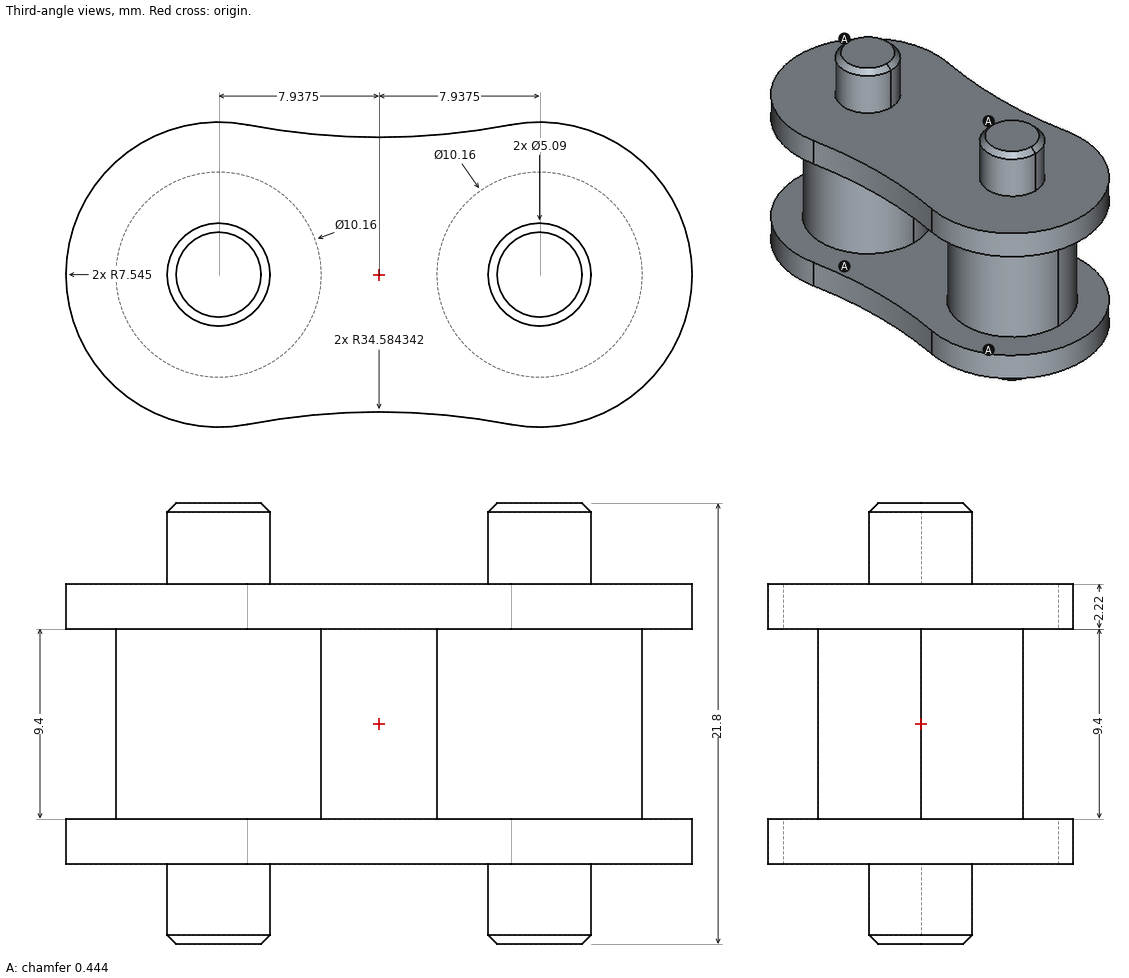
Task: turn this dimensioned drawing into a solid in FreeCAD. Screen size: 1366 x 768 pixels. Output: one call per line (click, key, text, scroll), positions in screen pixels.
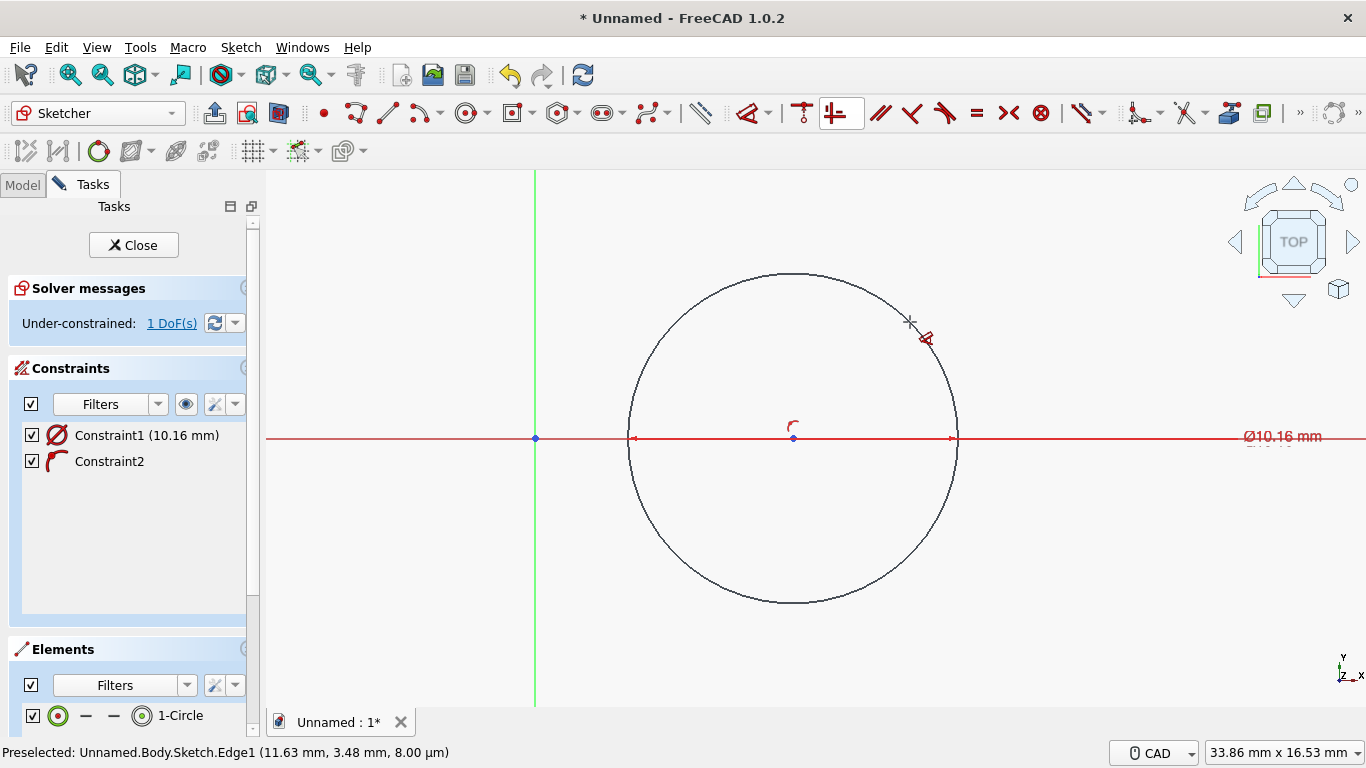
click(793, 438)
click(664, 472)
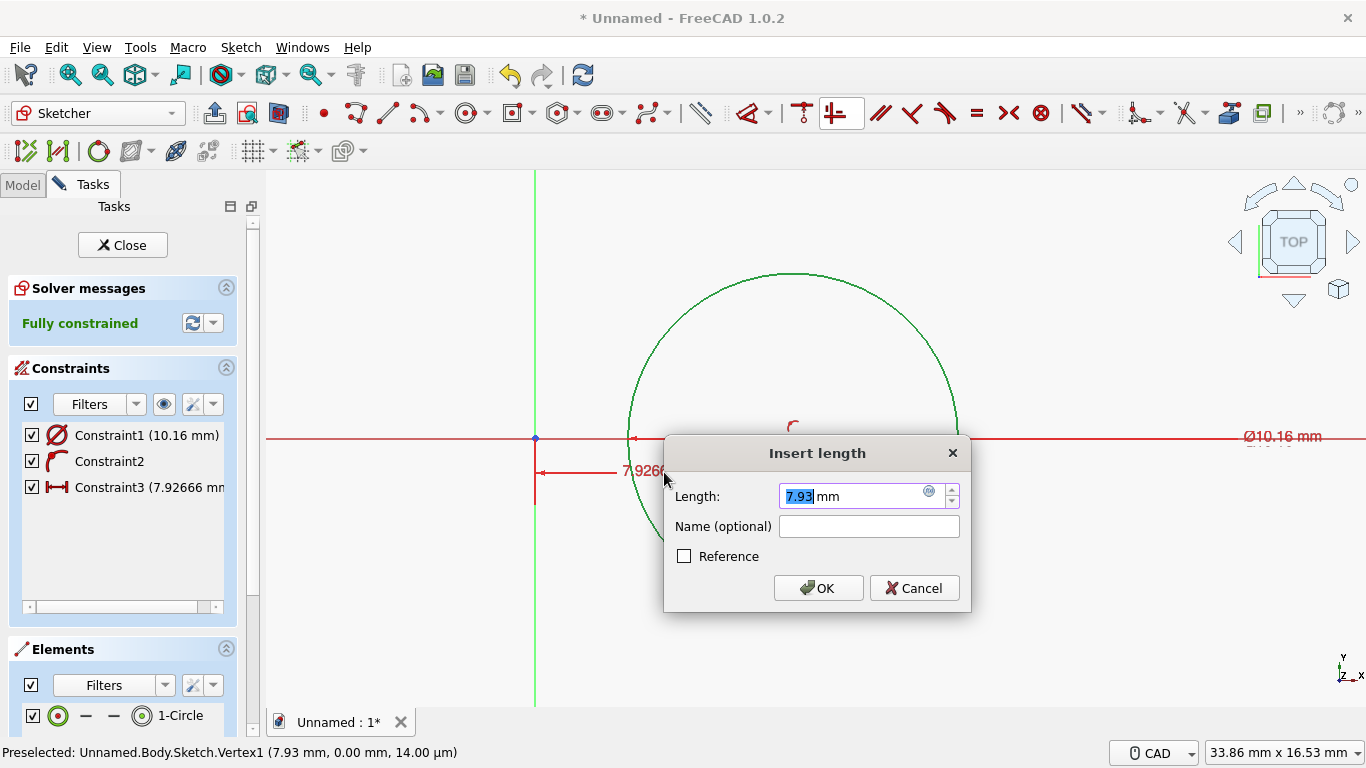
text(7.9375)
key(Return)
key(Escape)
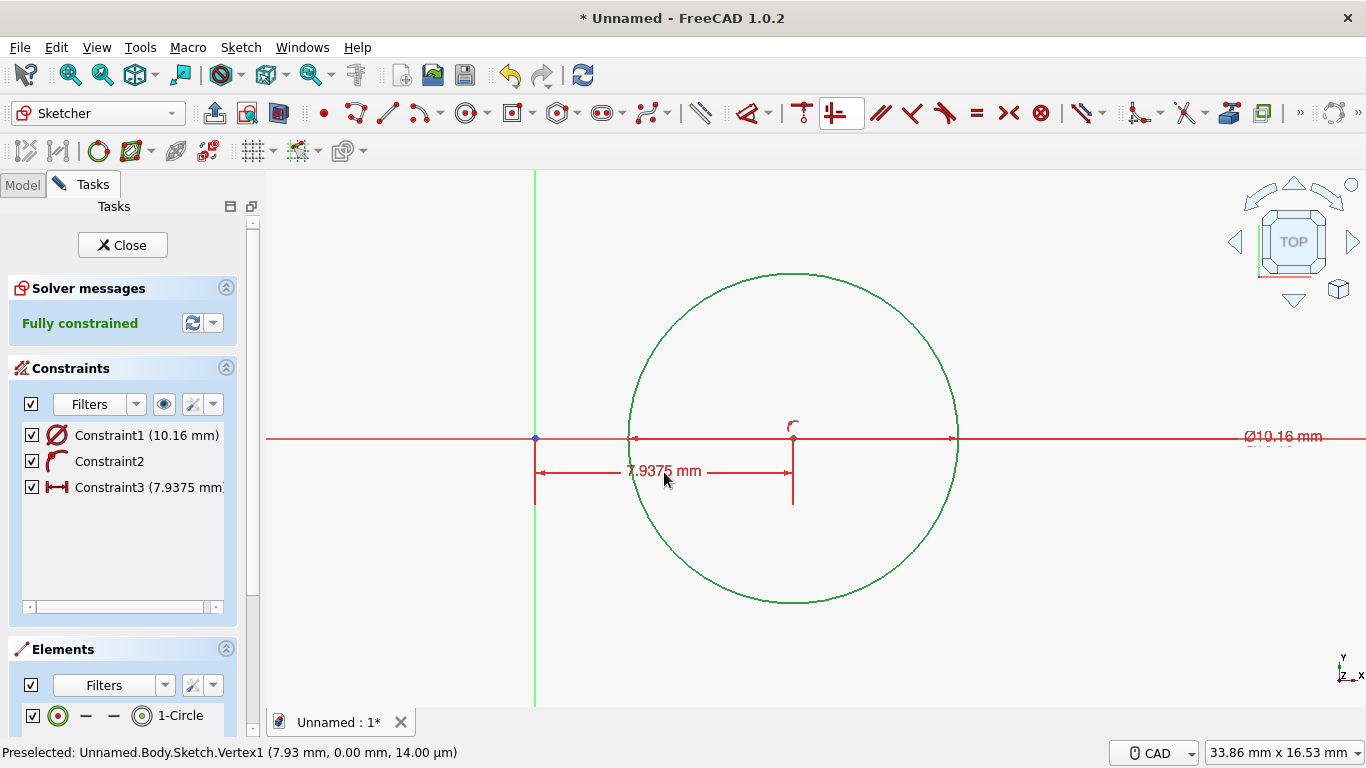
click(123, 245)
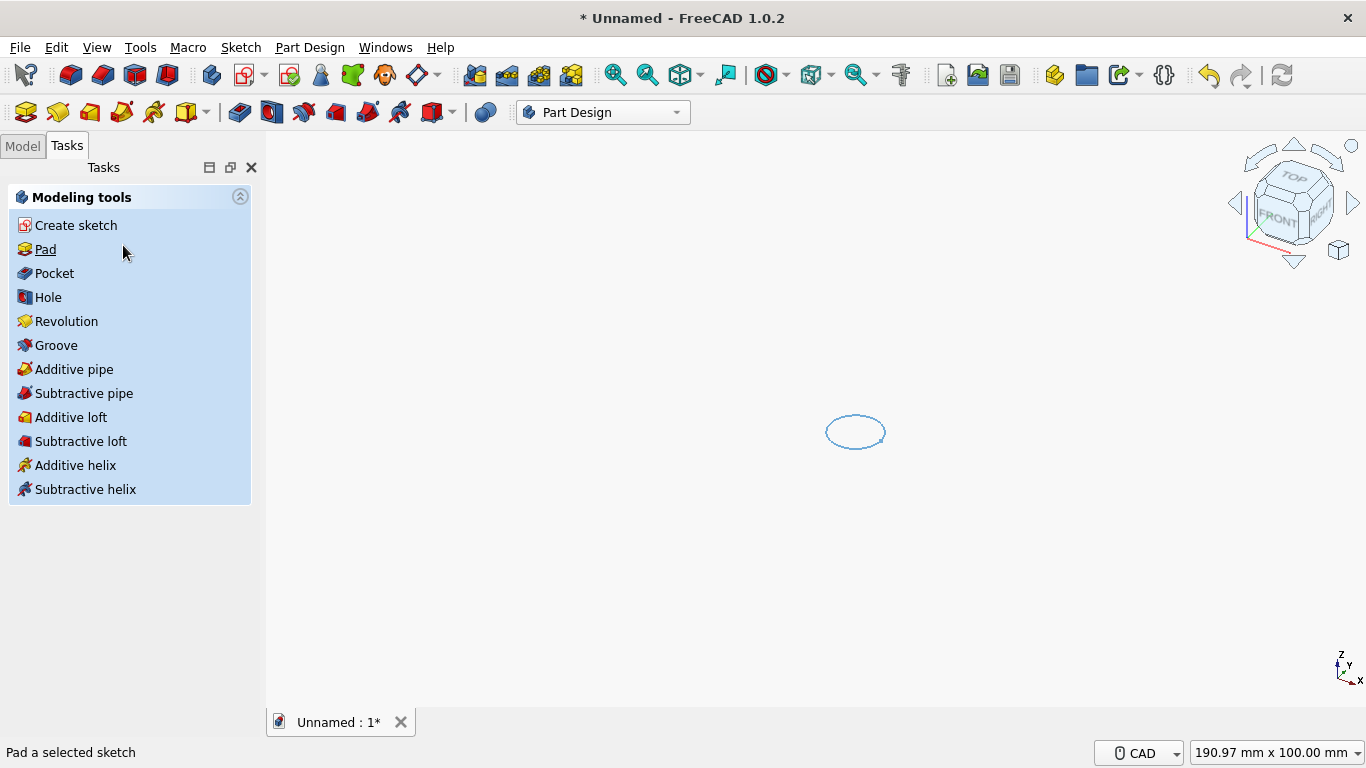
click(26, 112)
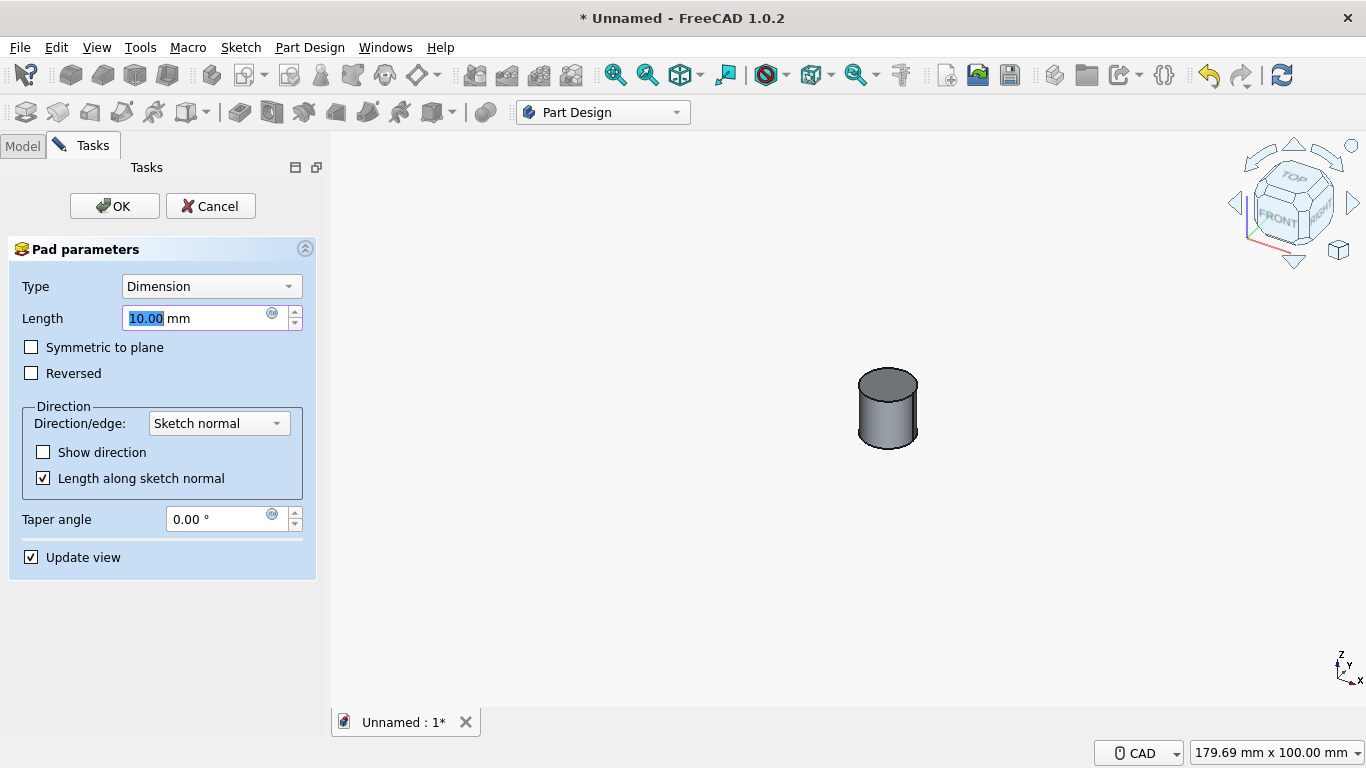
text(9.4)
key(Tab)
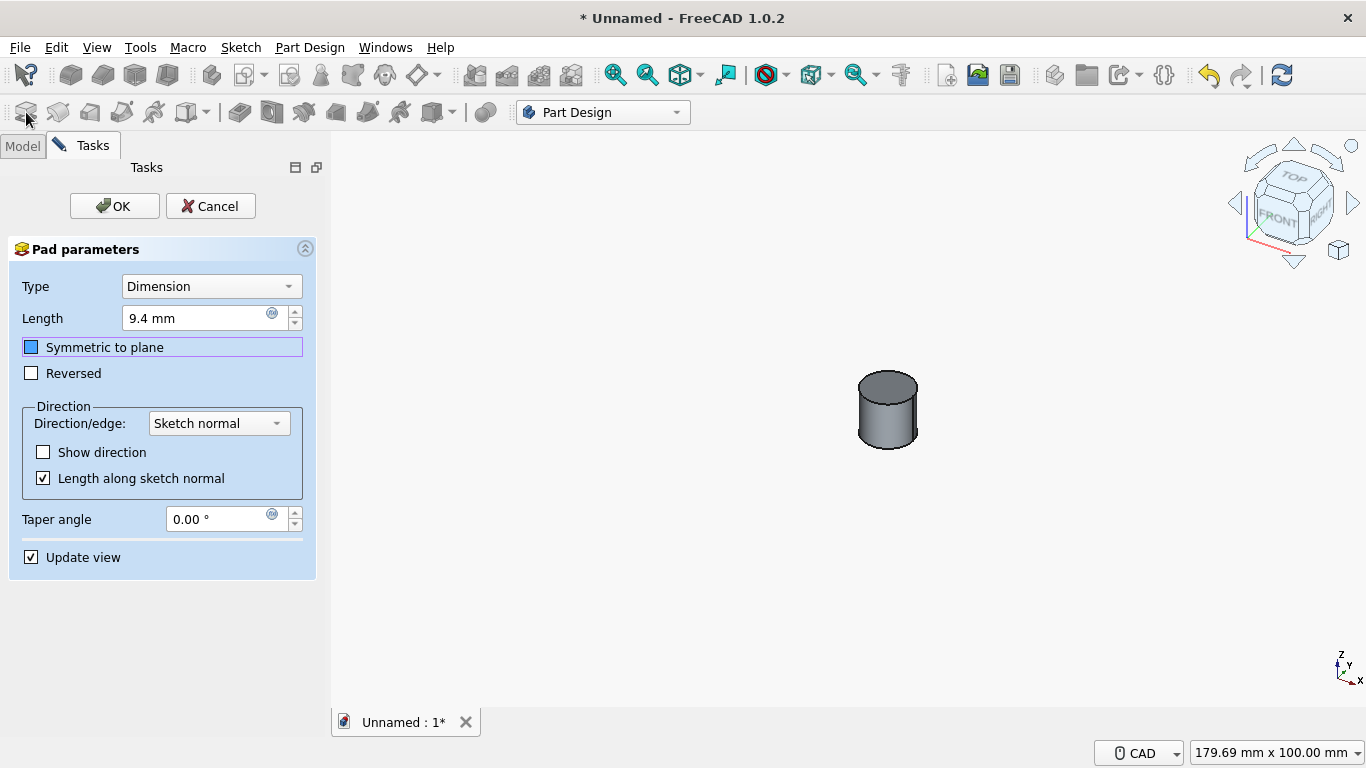
click(30, 347)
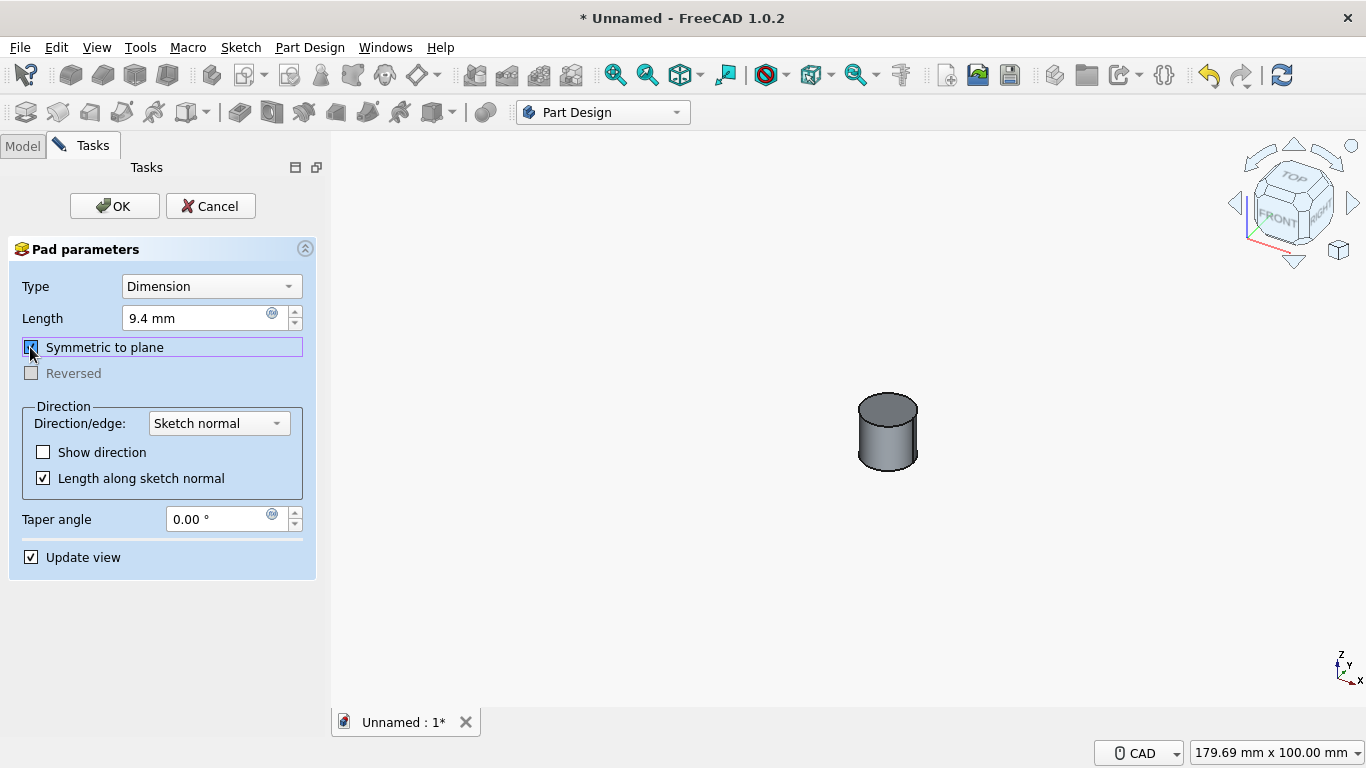
click(115, 206)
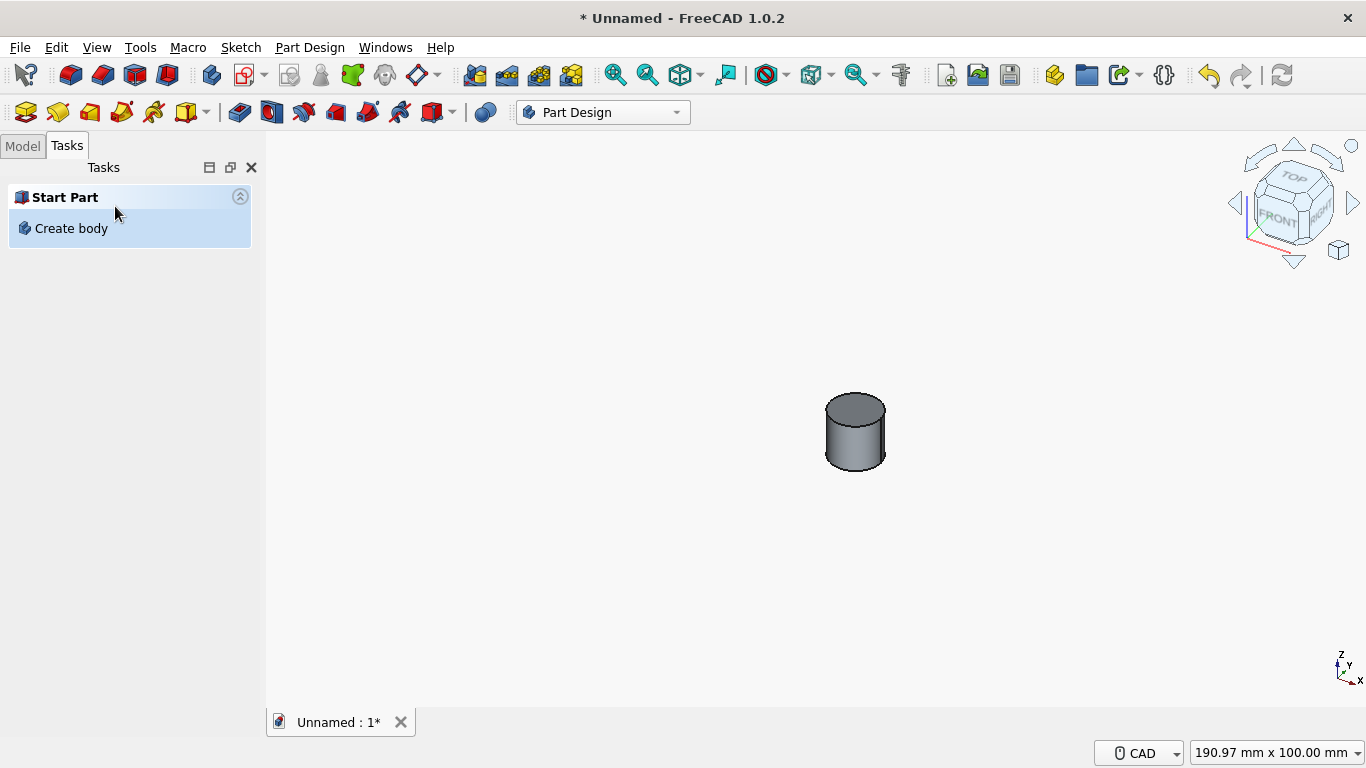
click(616, 76)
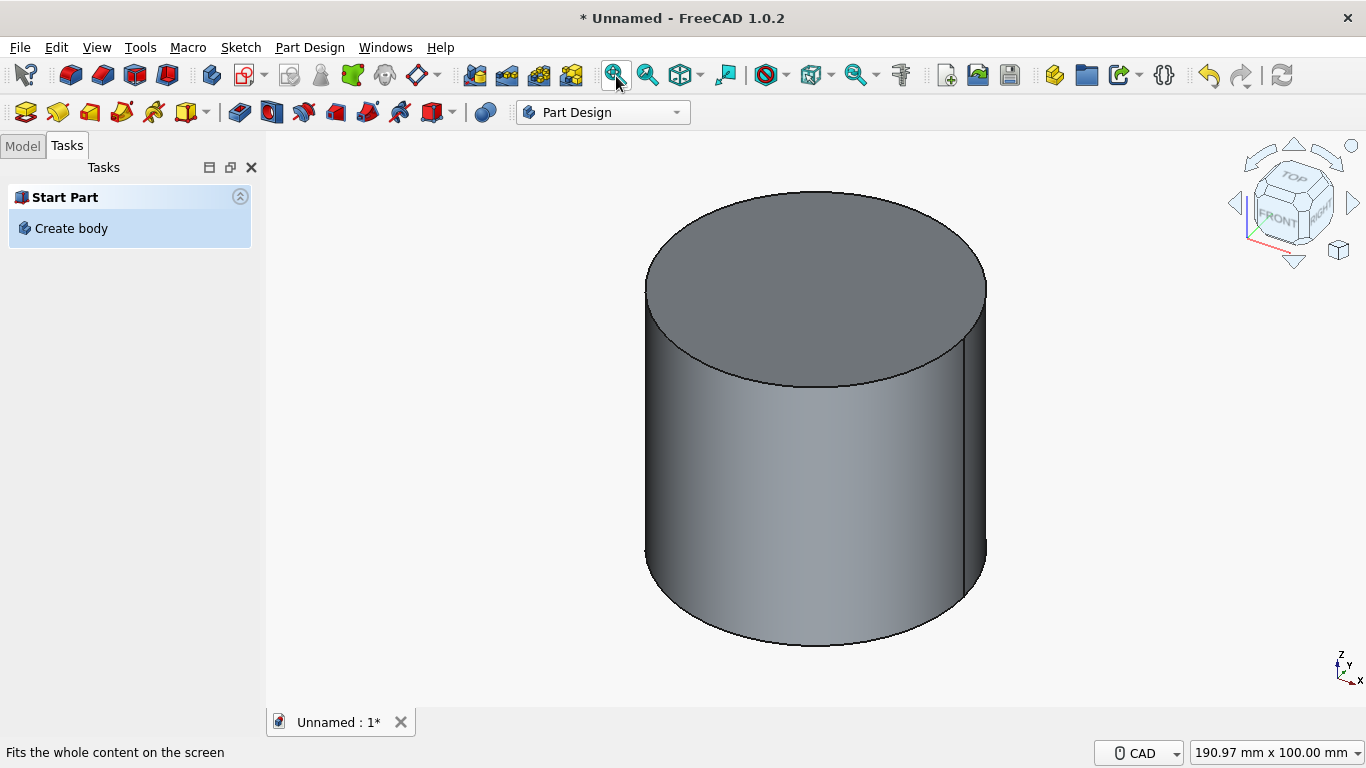
click(212, 76)